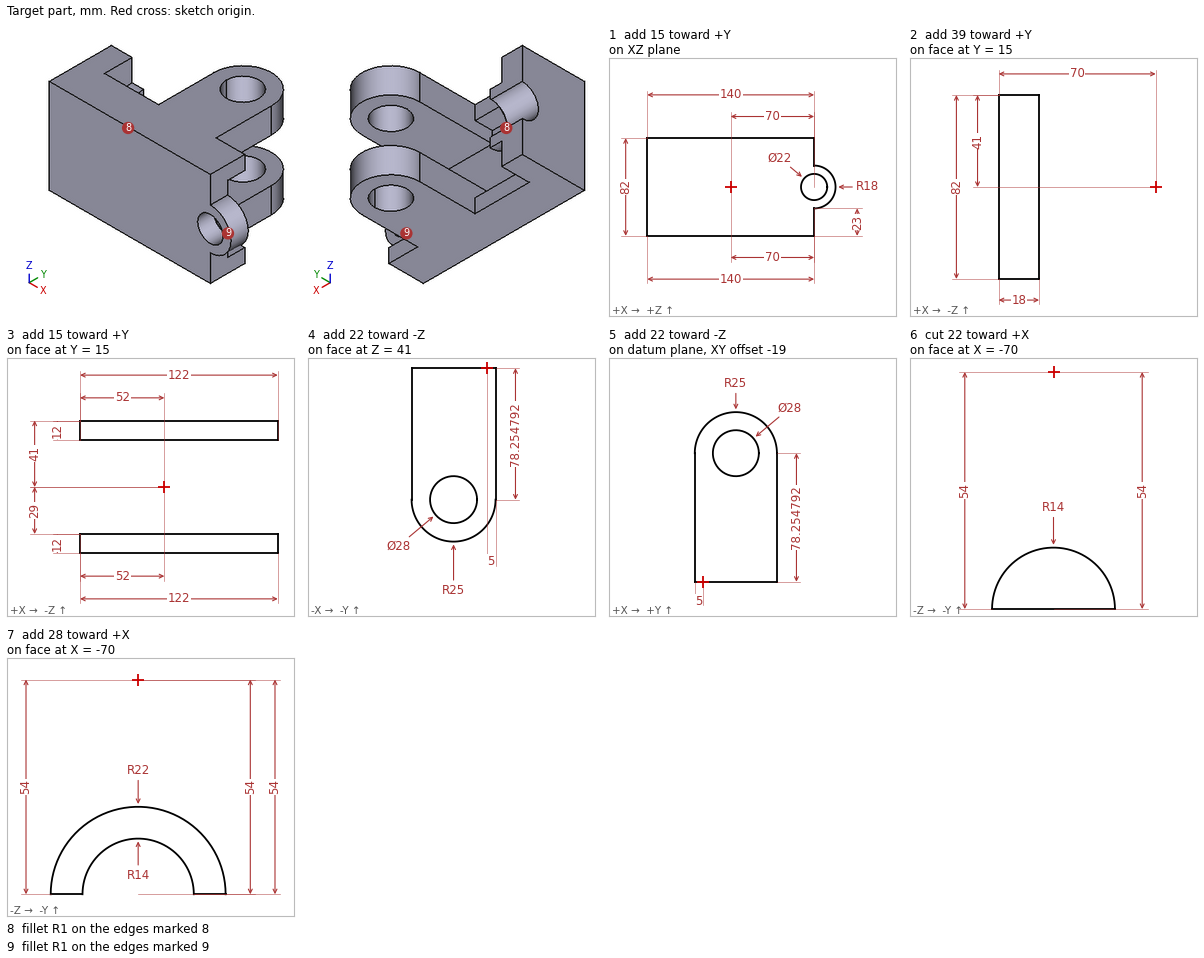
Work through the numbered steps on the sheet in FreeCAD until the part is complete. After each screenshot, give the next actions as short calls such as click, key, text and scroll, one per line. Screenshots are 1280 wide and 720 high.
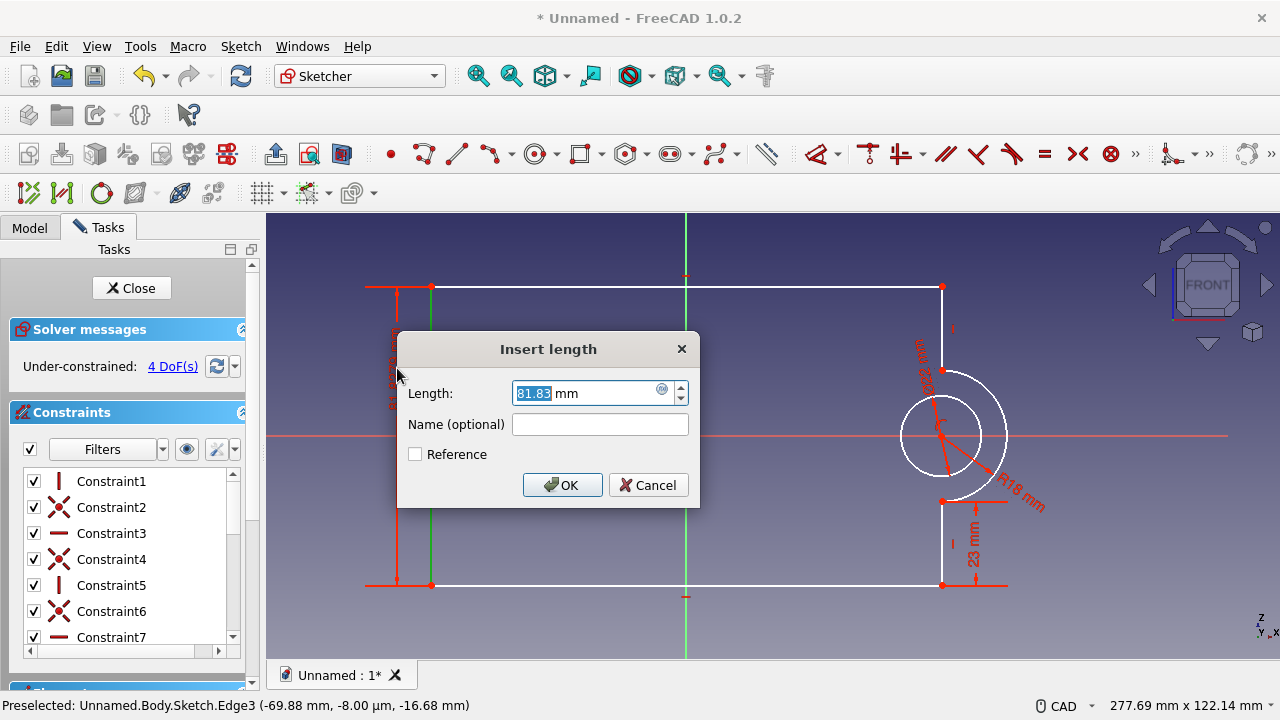
text(82)
key(Return)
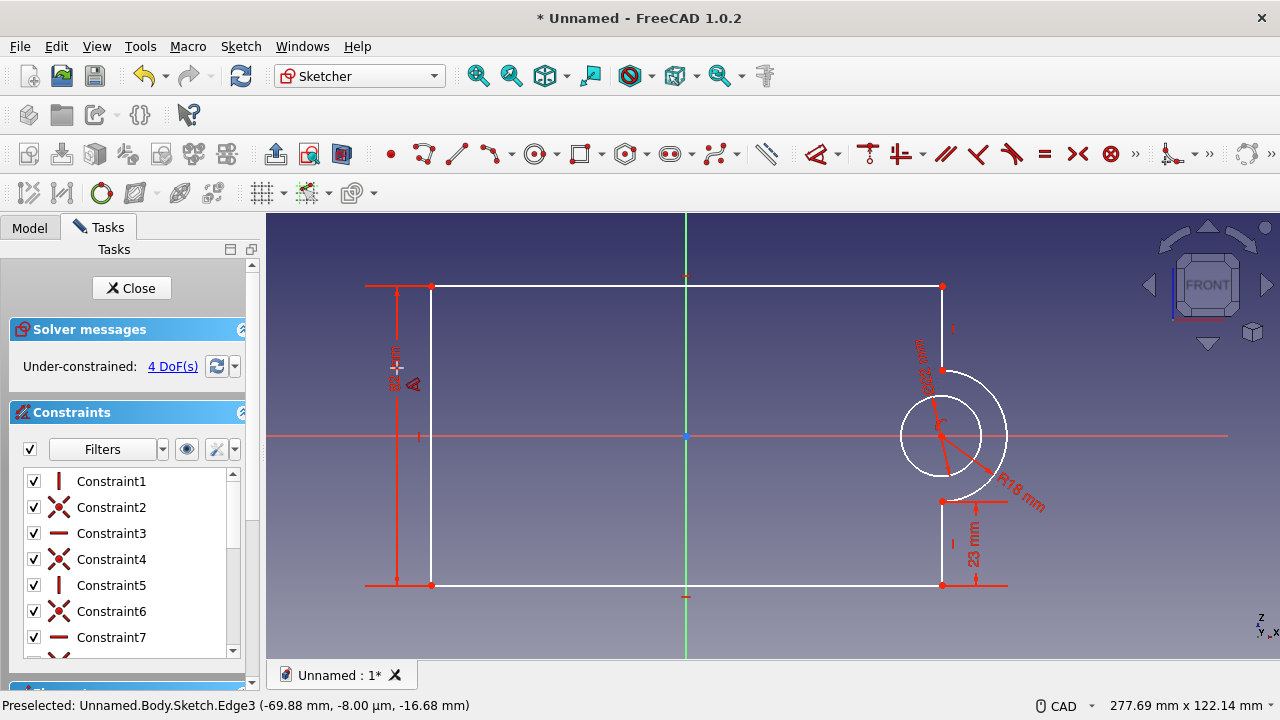
click(941, 436)
click(814, 470)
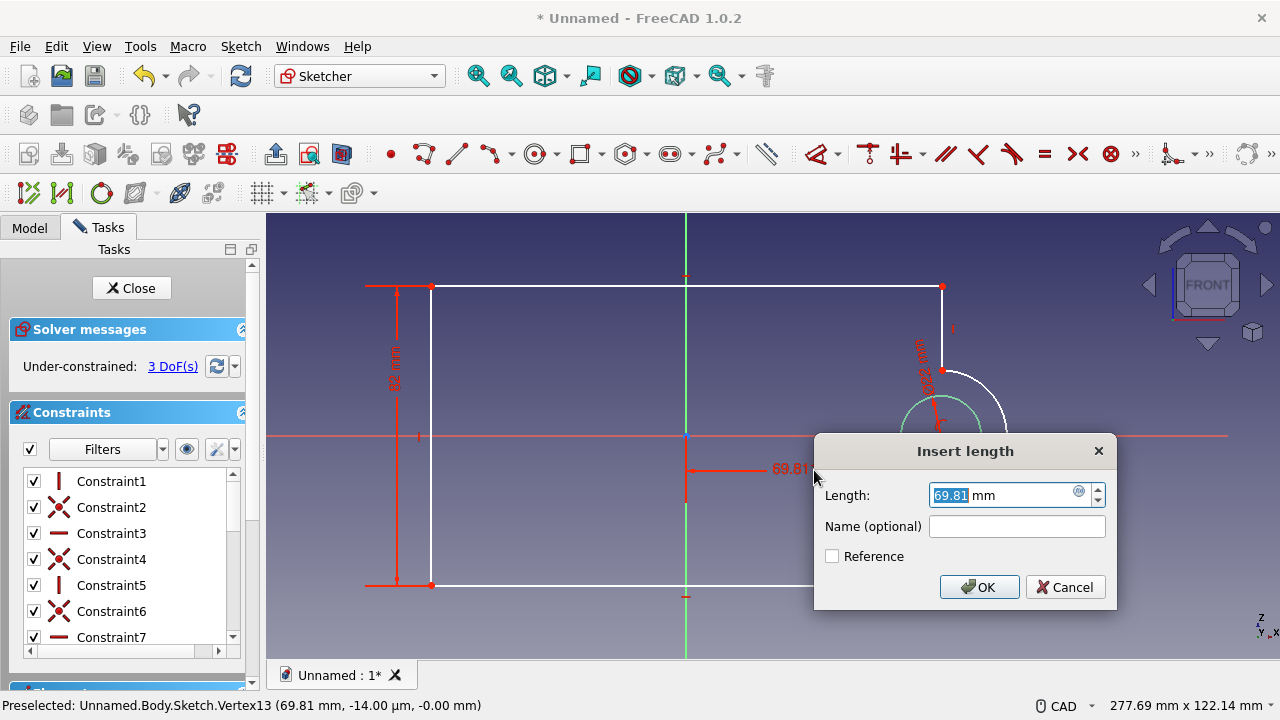
text(70)
key(Return)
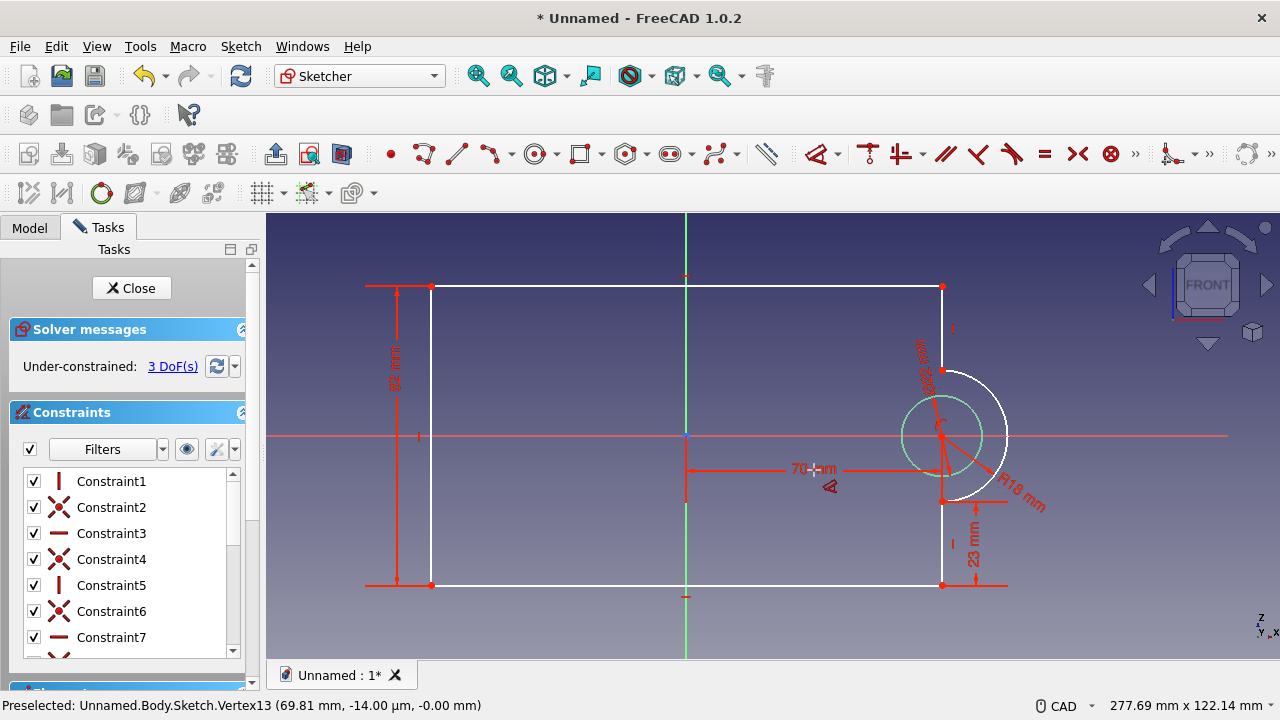
click(789, 586)
click(569, 620)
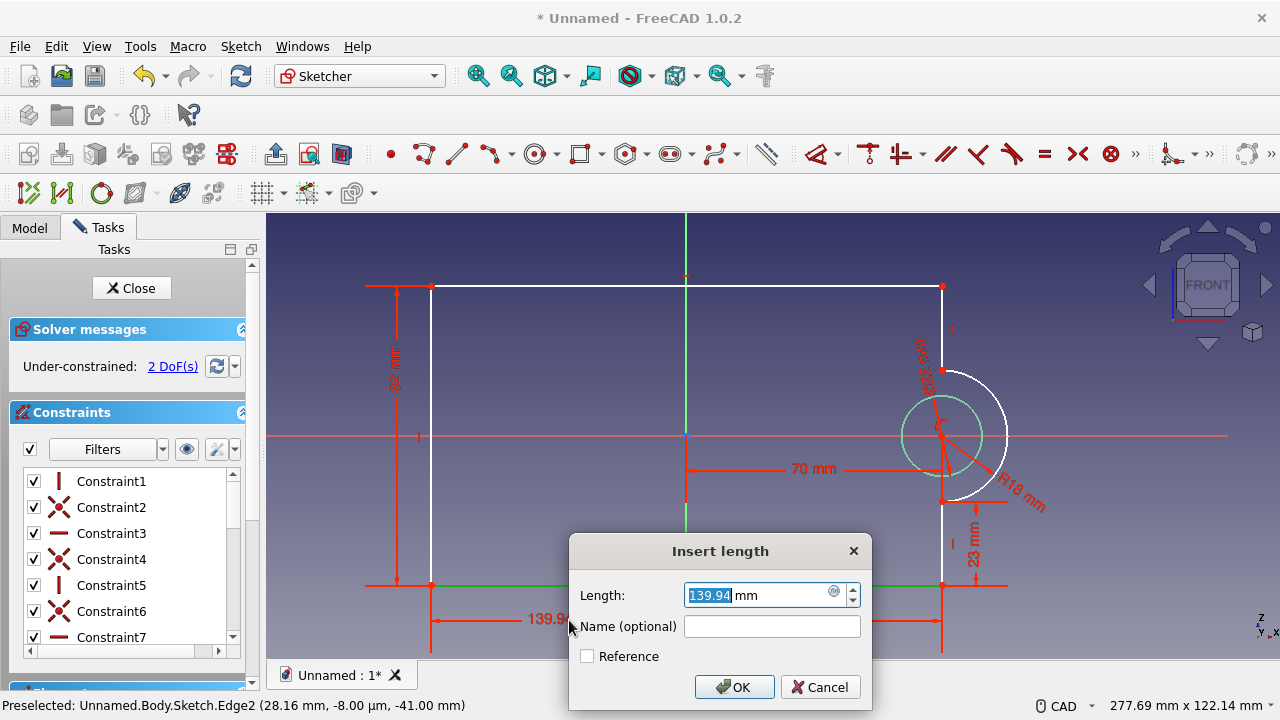
text(140)
key(Return)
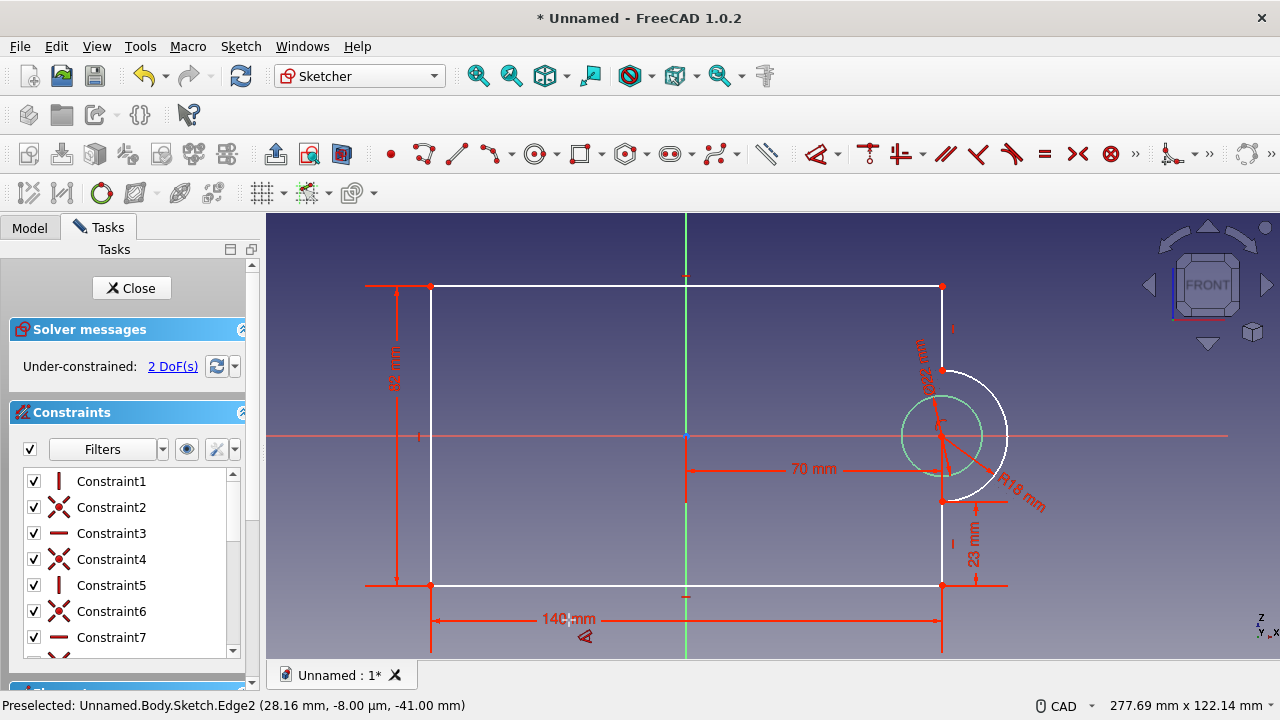
click(584, 286)
click(569, 252)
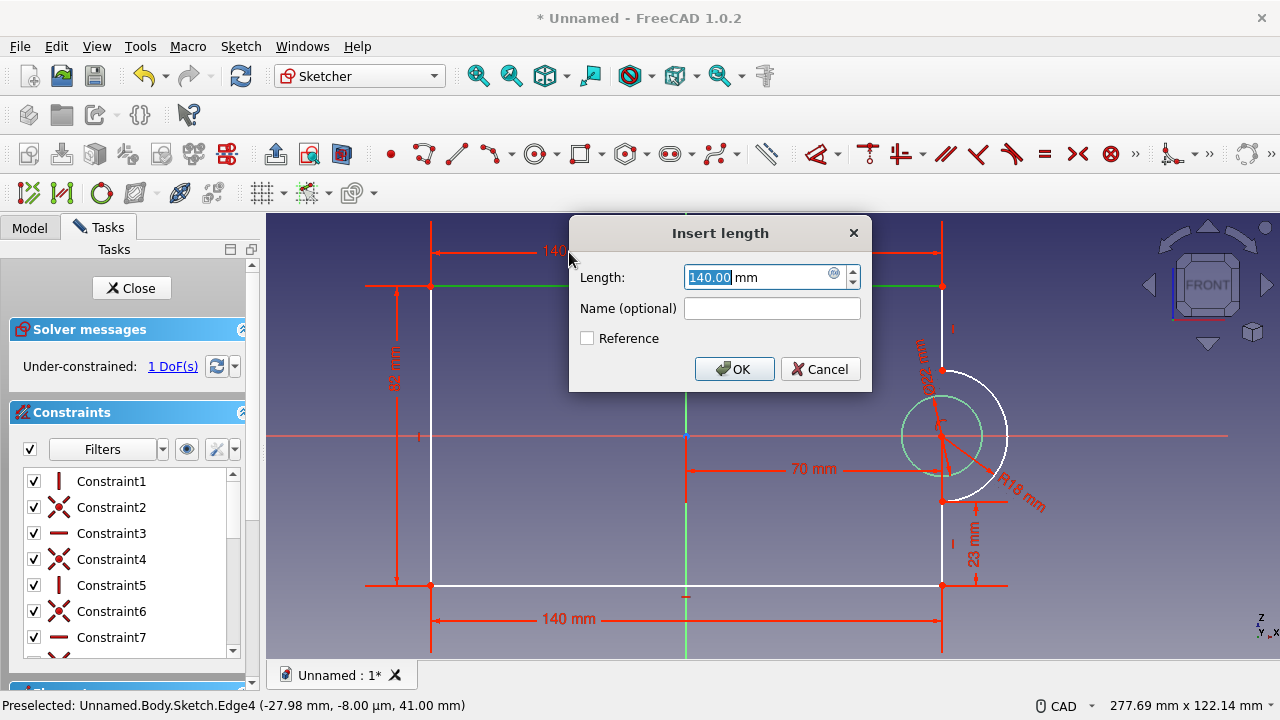
text(140)
key(Return)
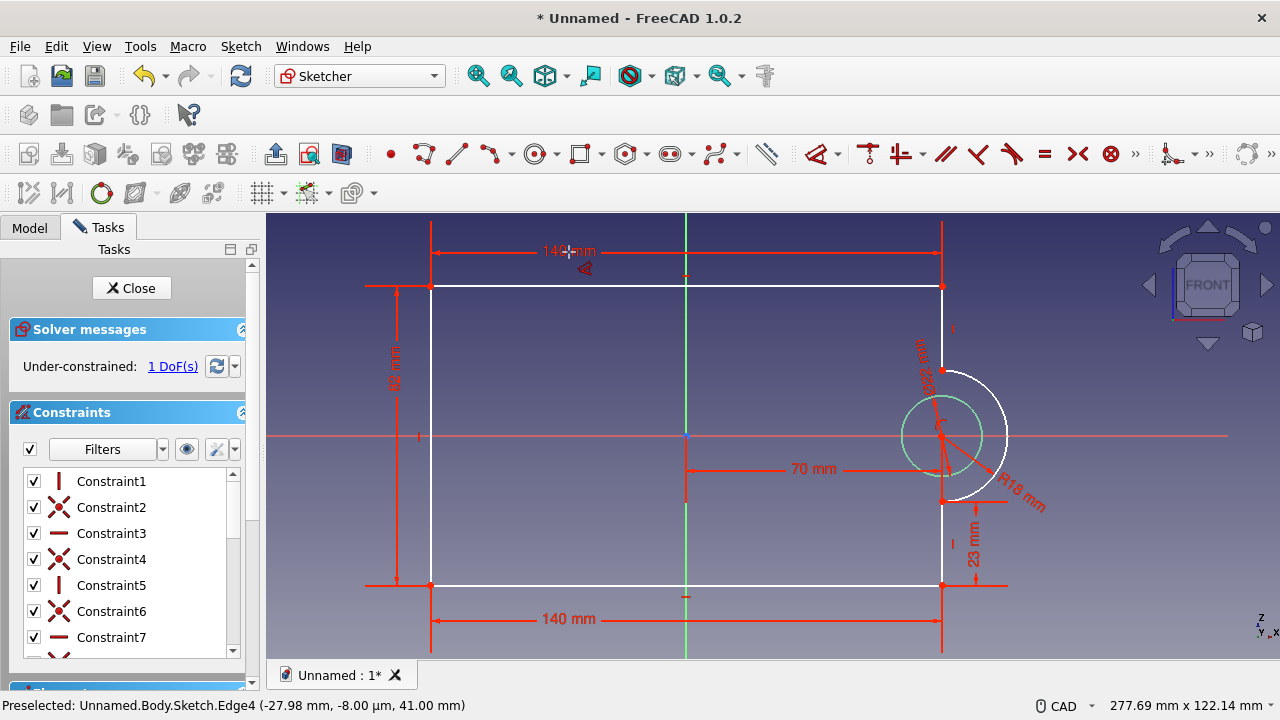
click(942, 502)
click(814, 536)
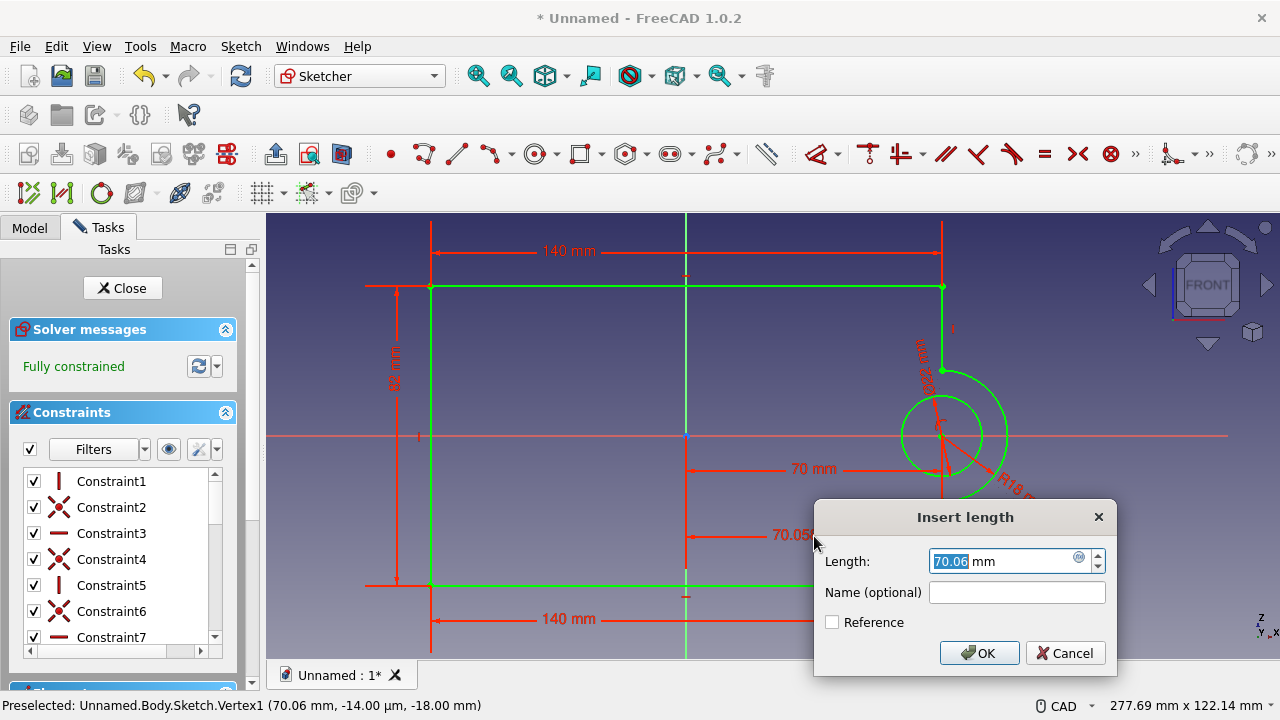
text(70)
key(Return)
key(Escape)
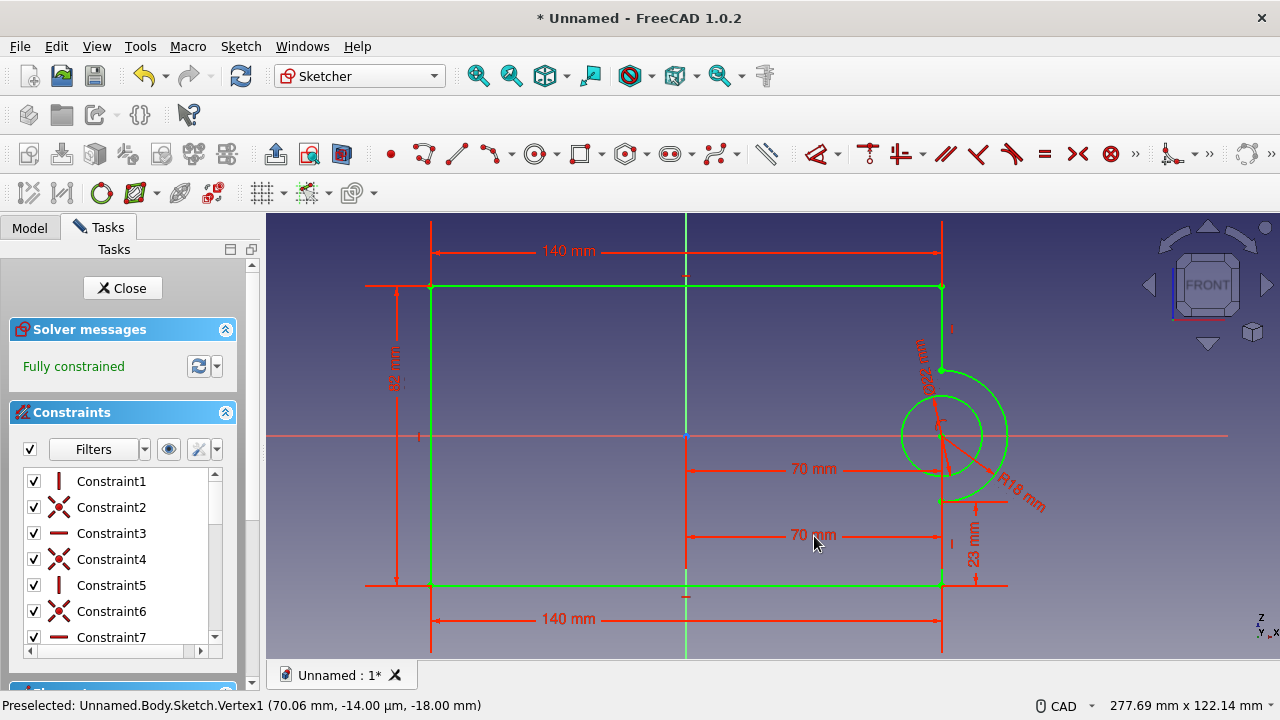
click(123, 288)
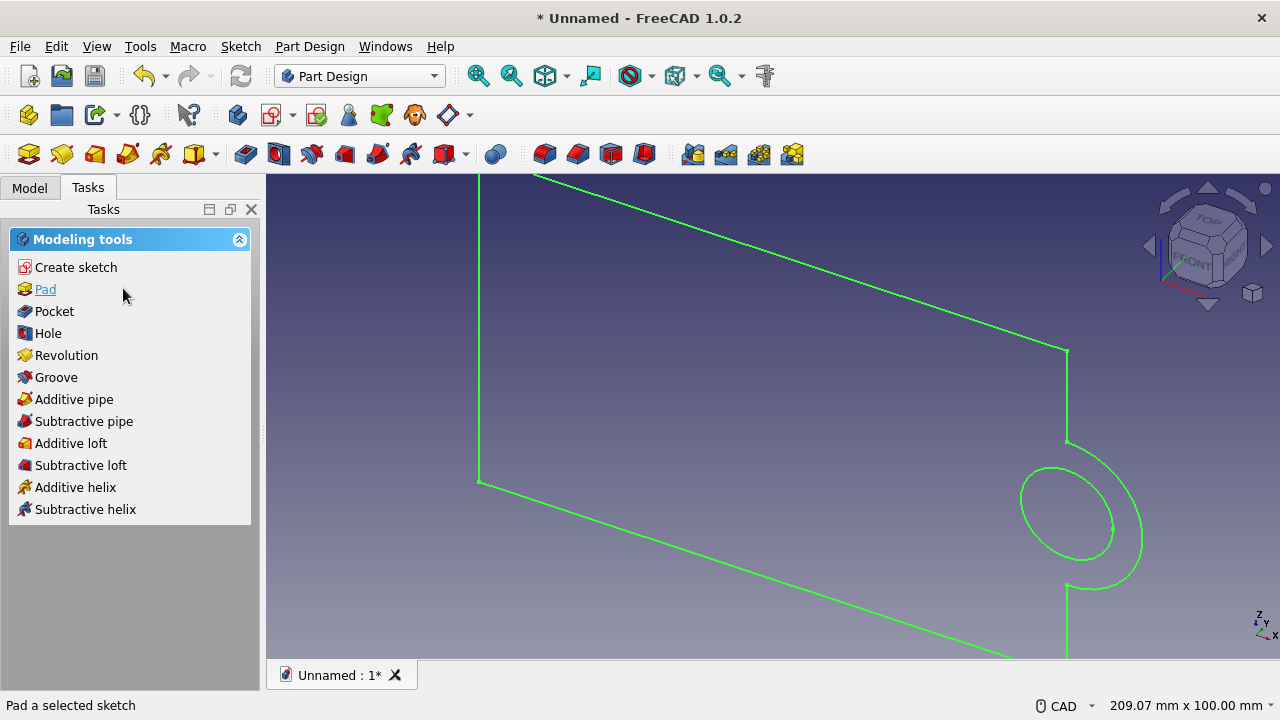
click(29, 154)